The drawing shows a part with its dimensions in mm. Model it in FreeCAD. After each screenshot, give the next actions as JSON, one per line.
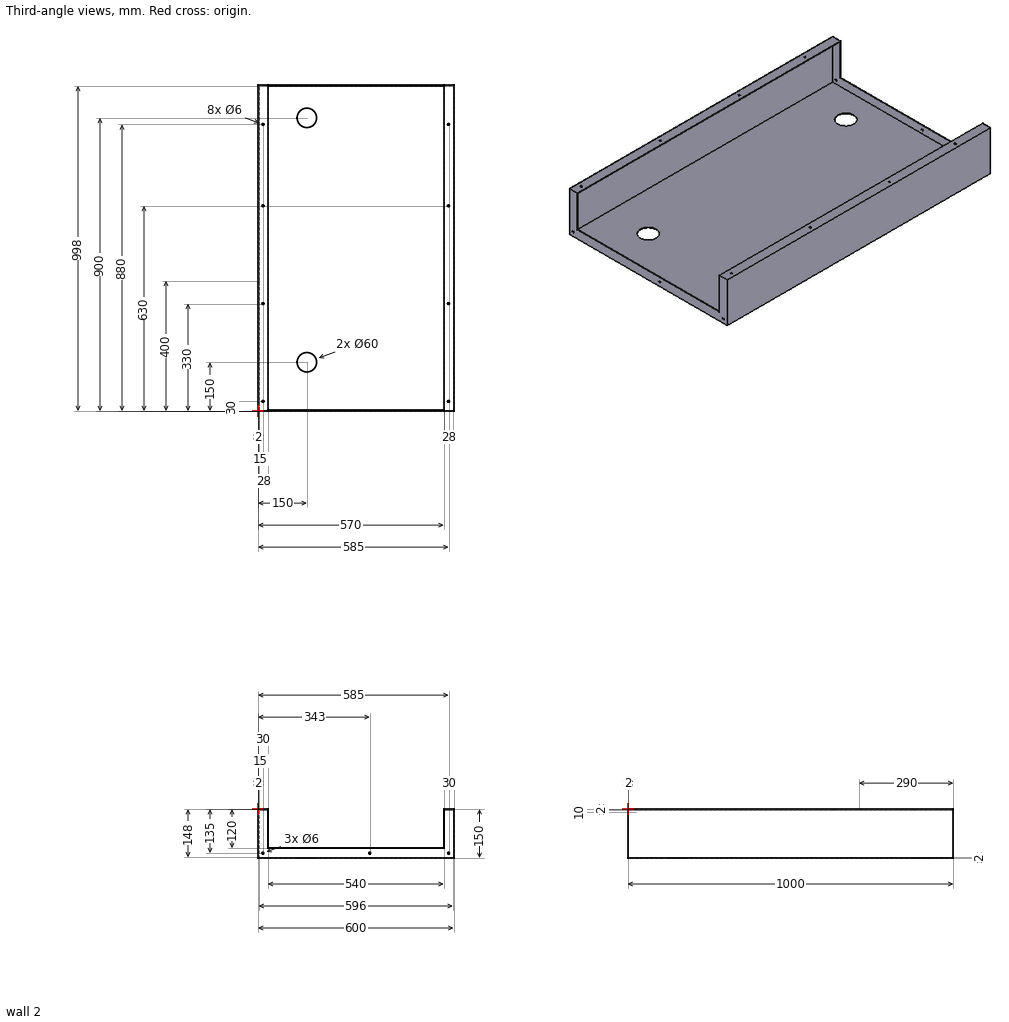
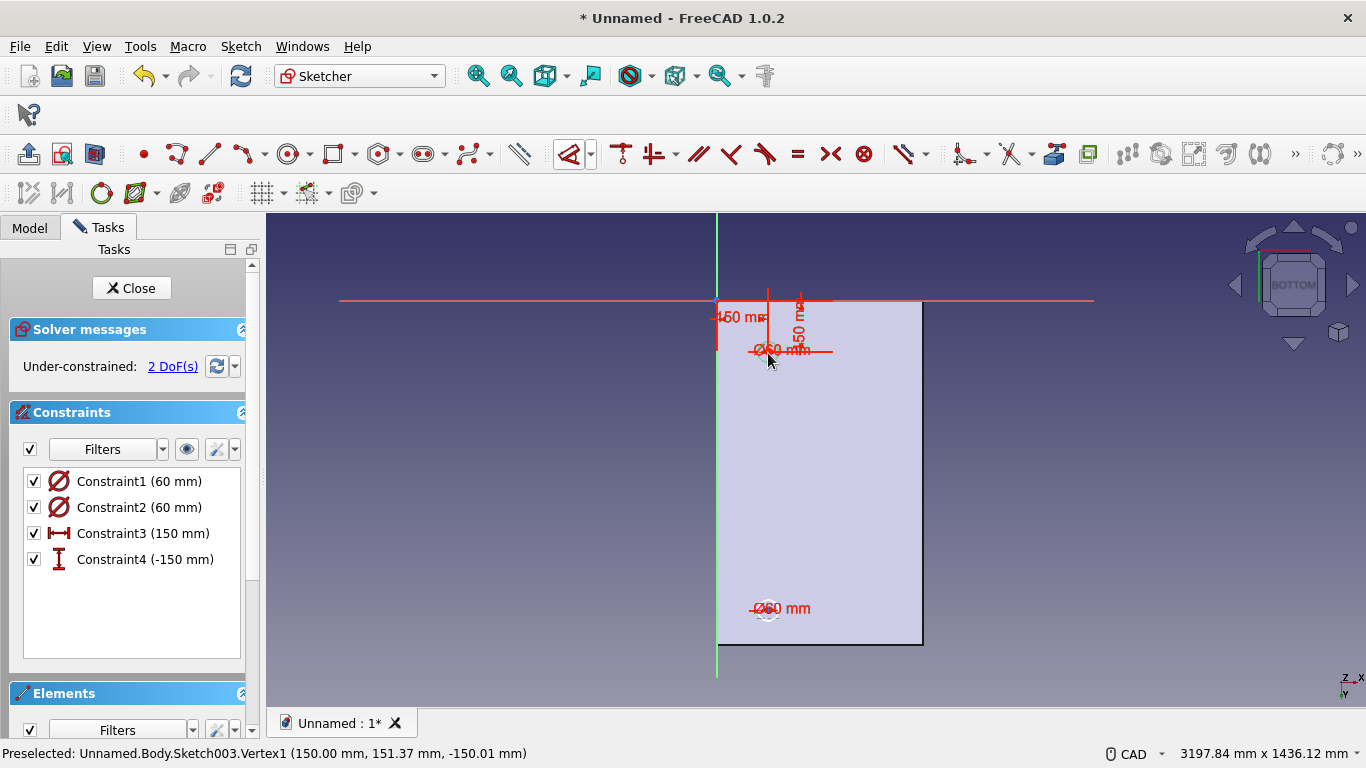
{"action": "left_click", "coordinate": [768, 611]}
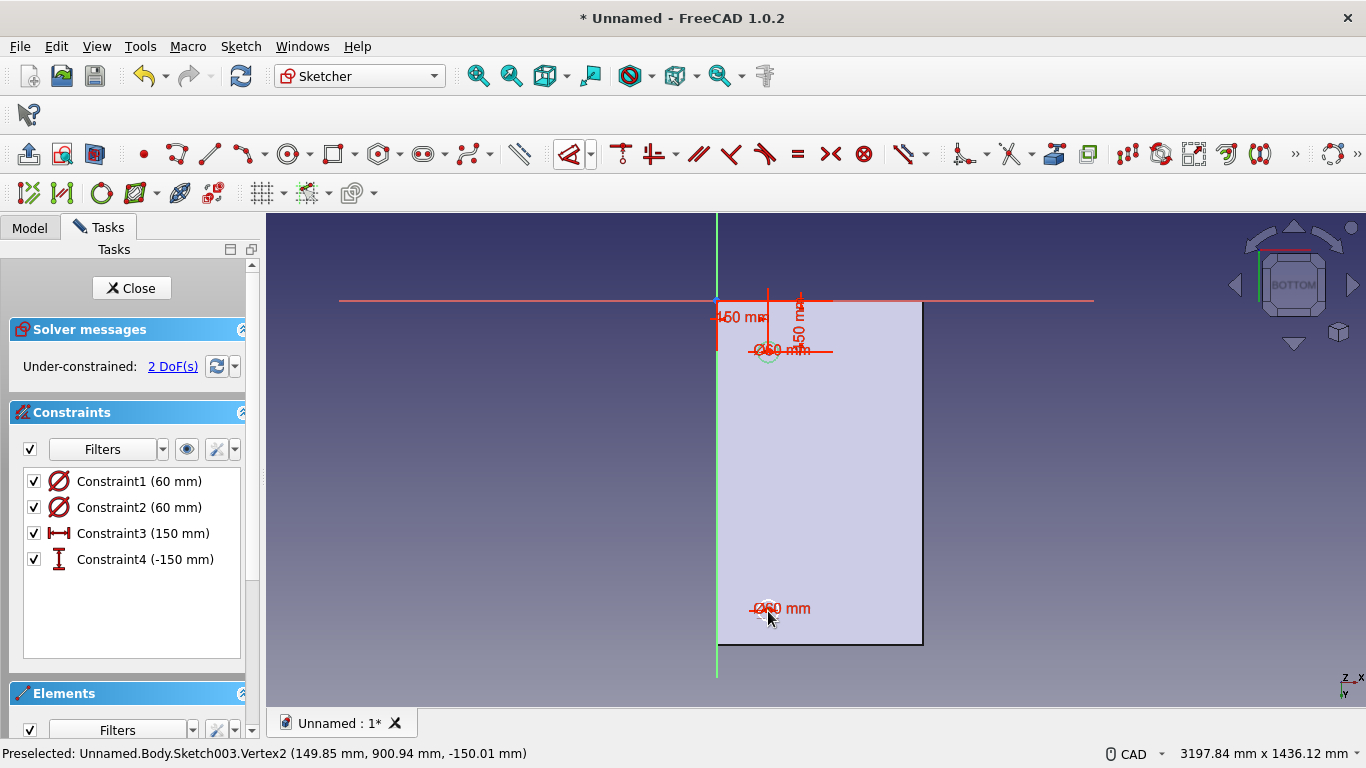
{"action": "key", "text": "l"}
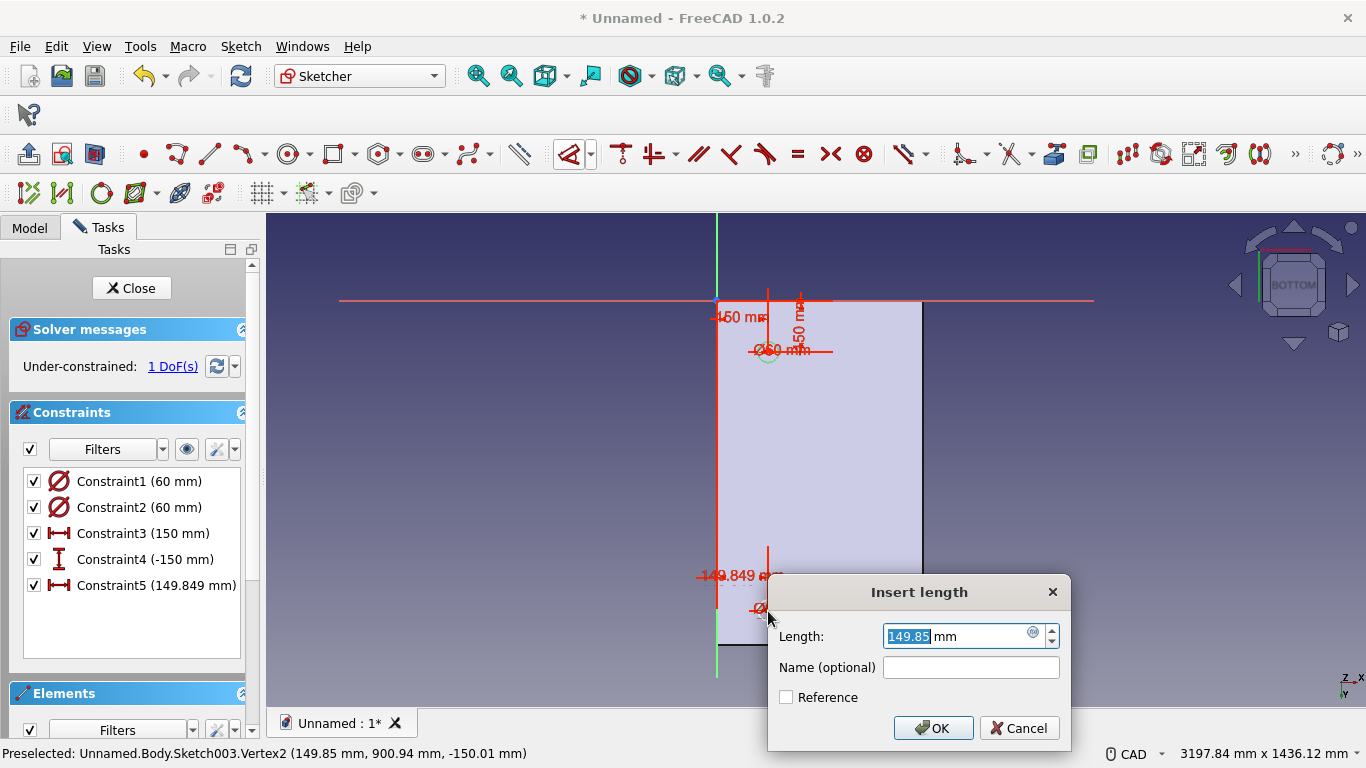
{"action": "type", "text": "150"}
{"action": "key", "text": "Return"}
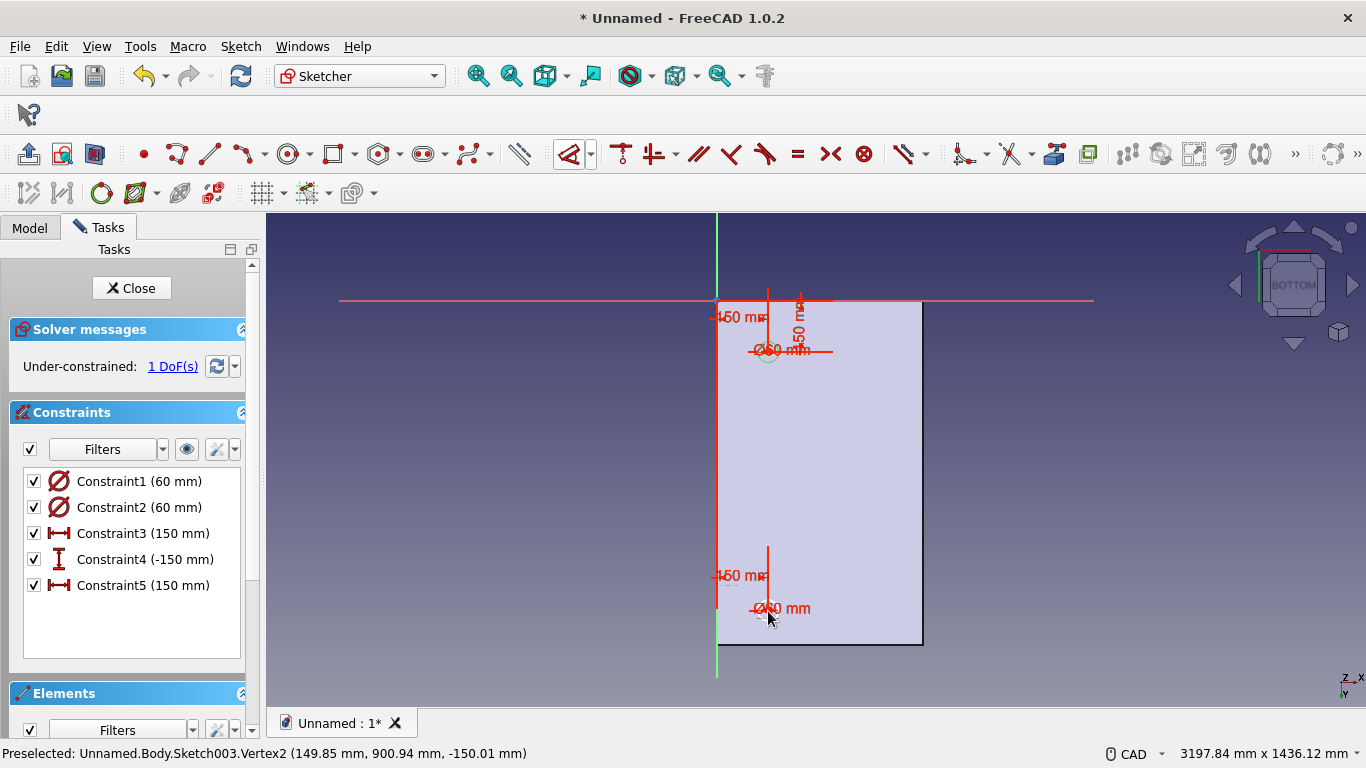
{"action": "left_click", "coordinate": [768, 611]}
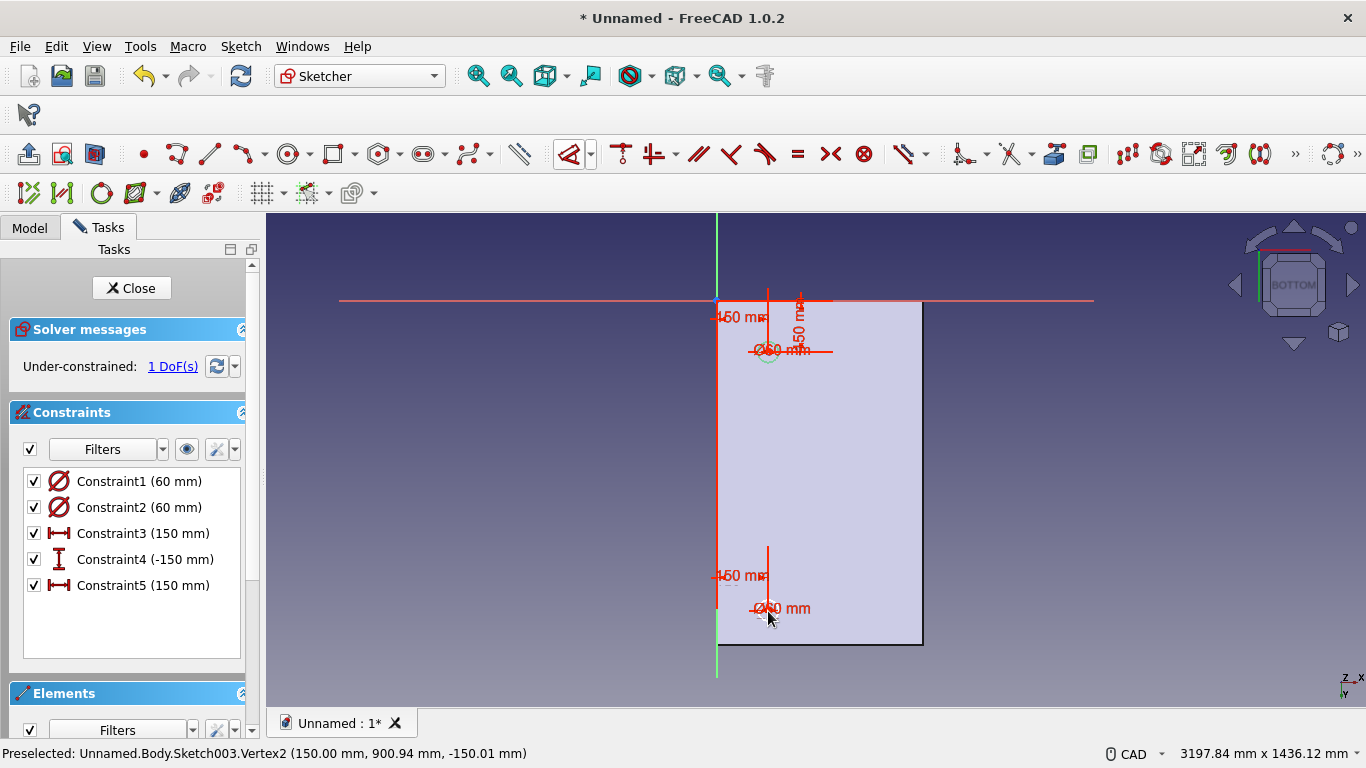
{"action": "key", "text": "i"}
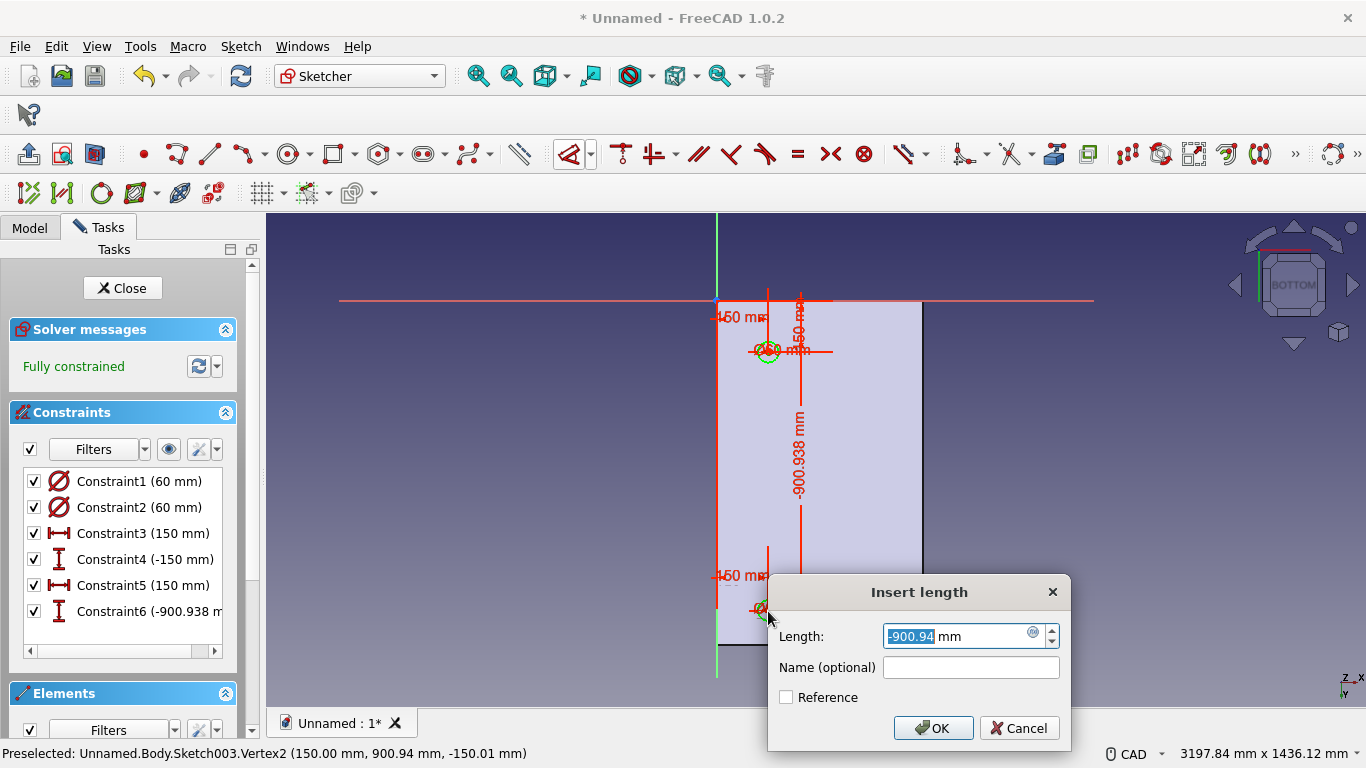
{"action": "type", "text": "-900"}
{"action": "key", "text": "Return"}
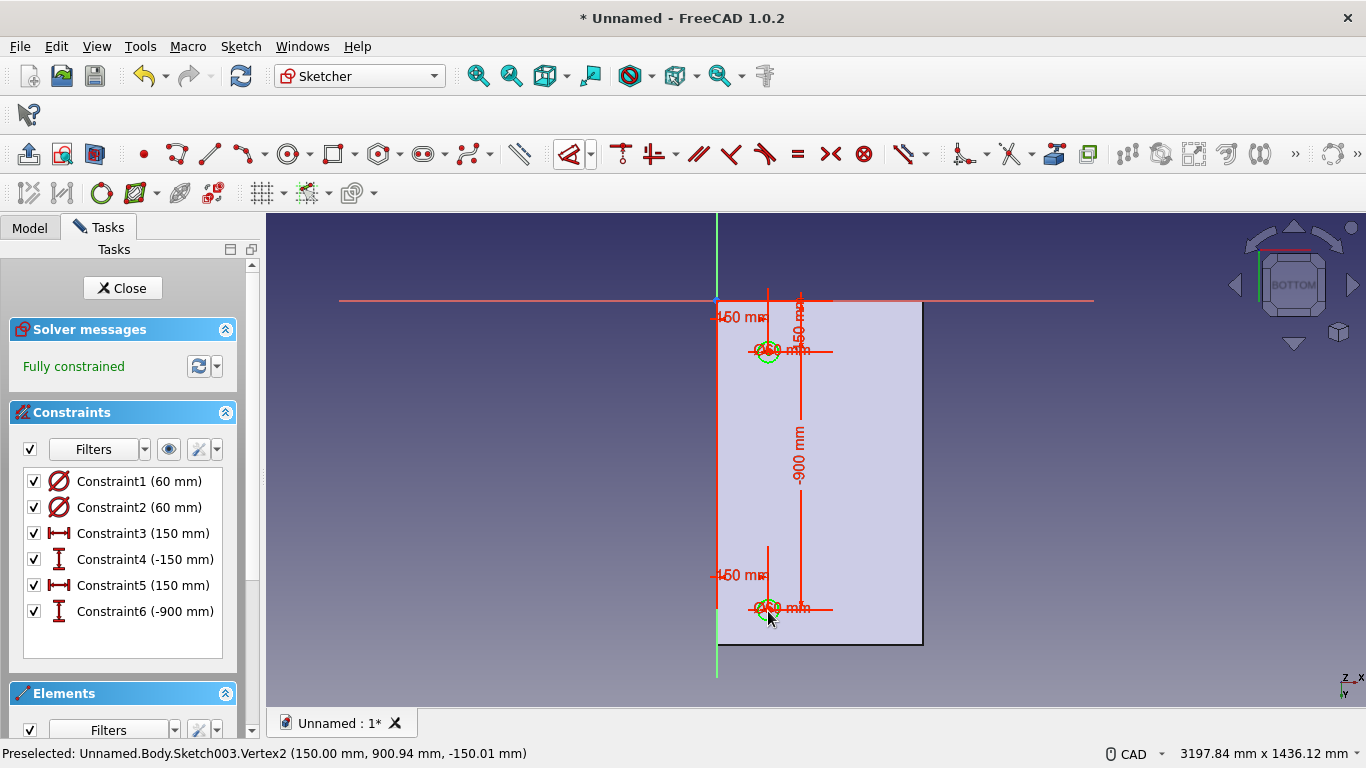
{"action": "left_click", "coordinate": [123, 288]}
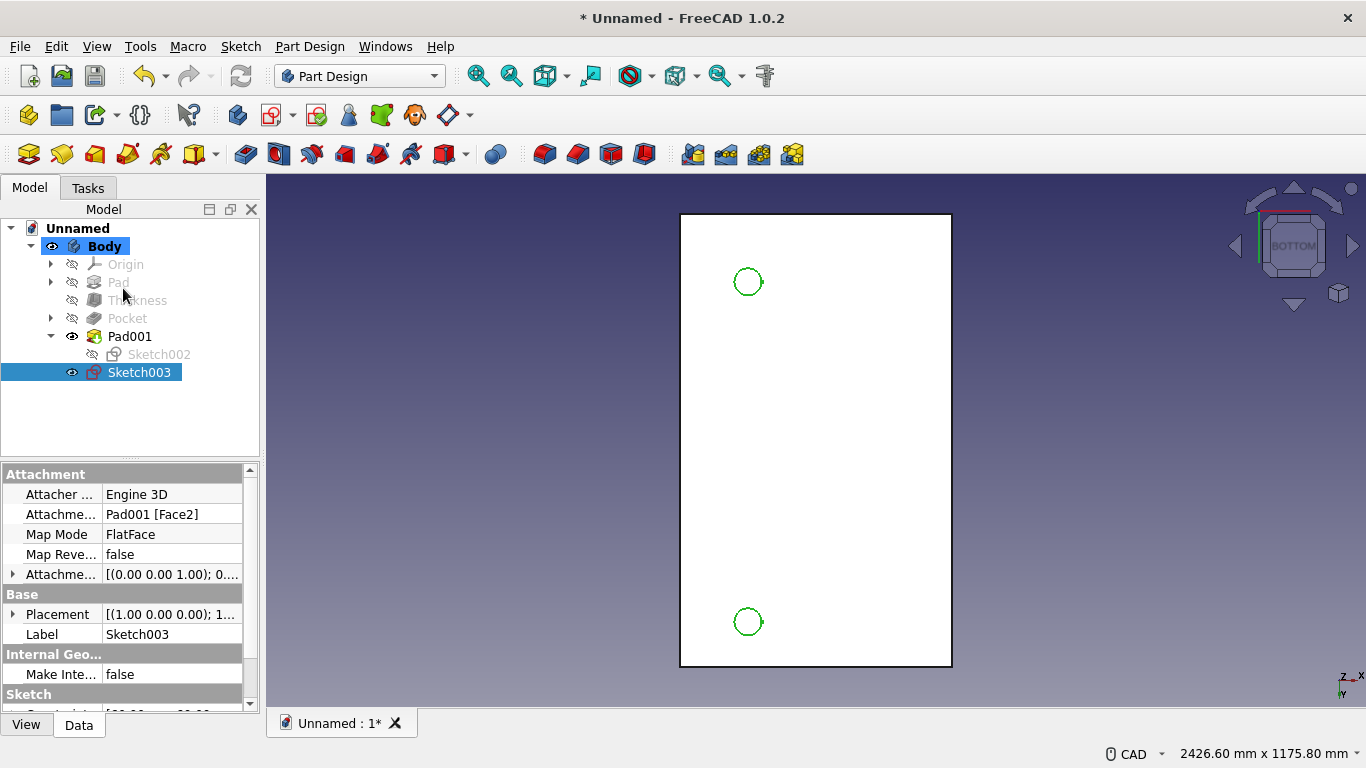
{"action": "left_click", "coordinate": [246, 154]}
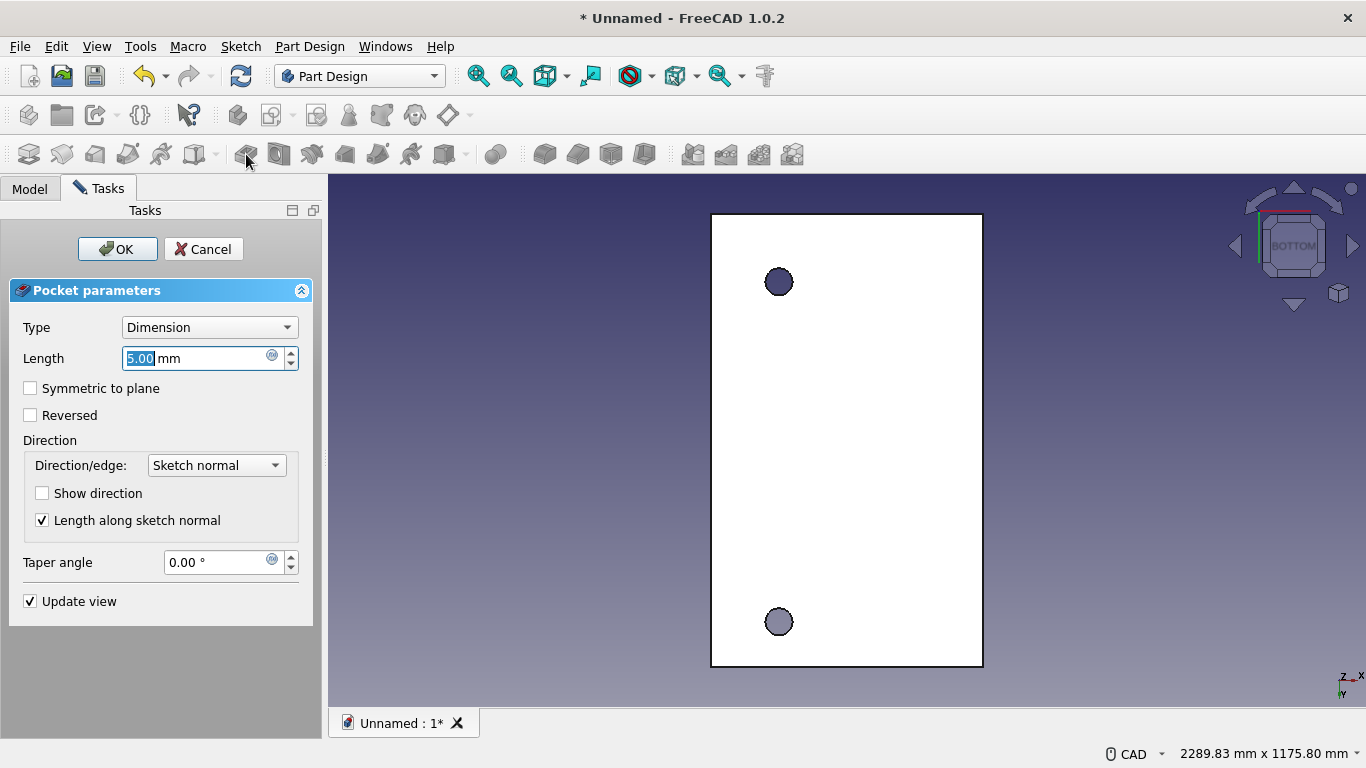
{"action": "type", "text": "2"}
{"action": "key", "text": "Tab"}